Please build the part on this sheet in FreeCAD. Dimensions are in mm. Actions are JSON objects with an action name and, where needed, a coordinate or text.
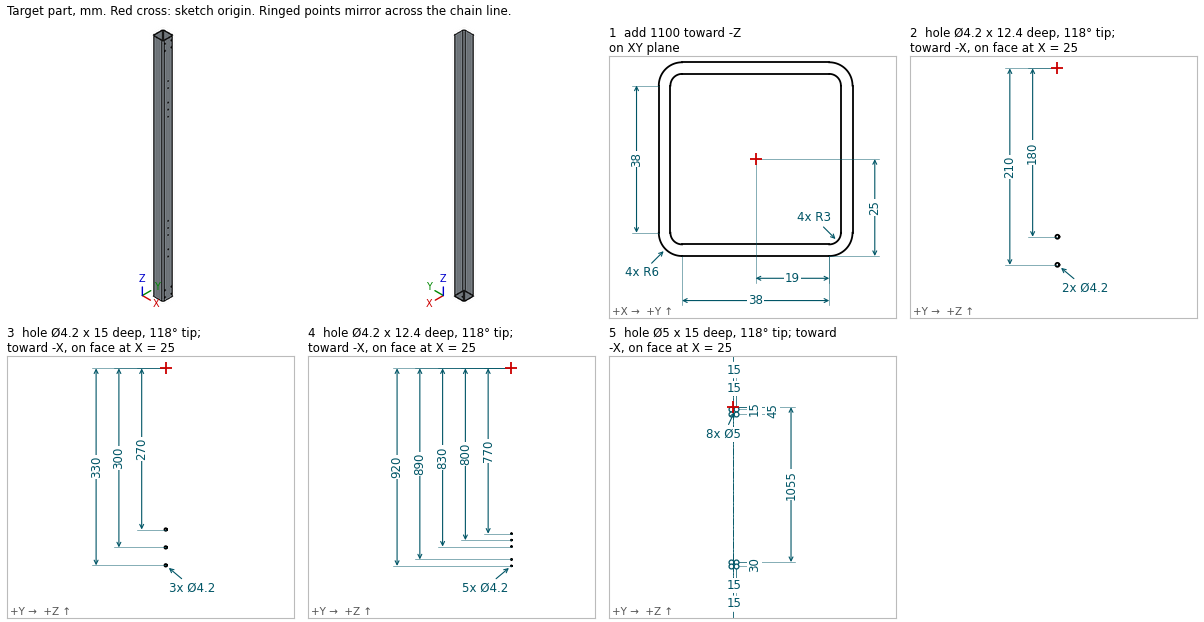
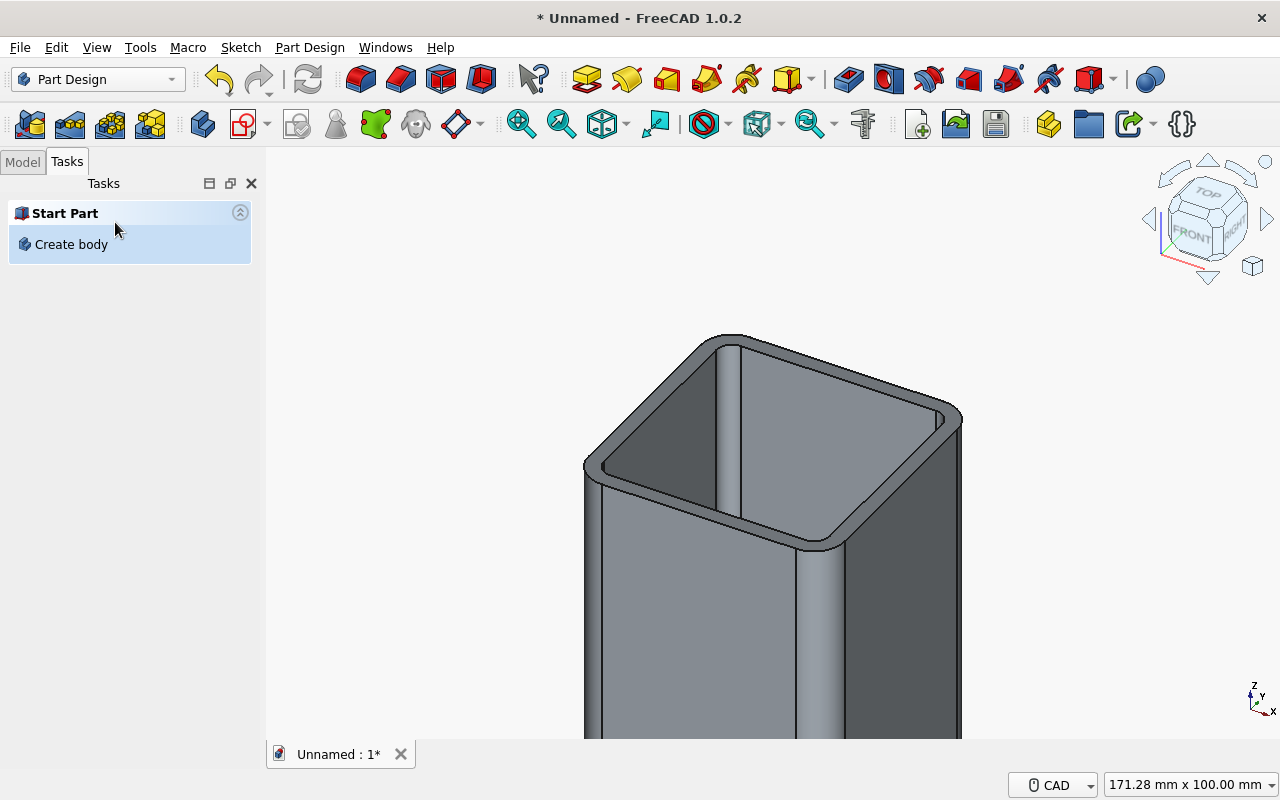
{"action": "left_click", "coordinate": [522, 124]}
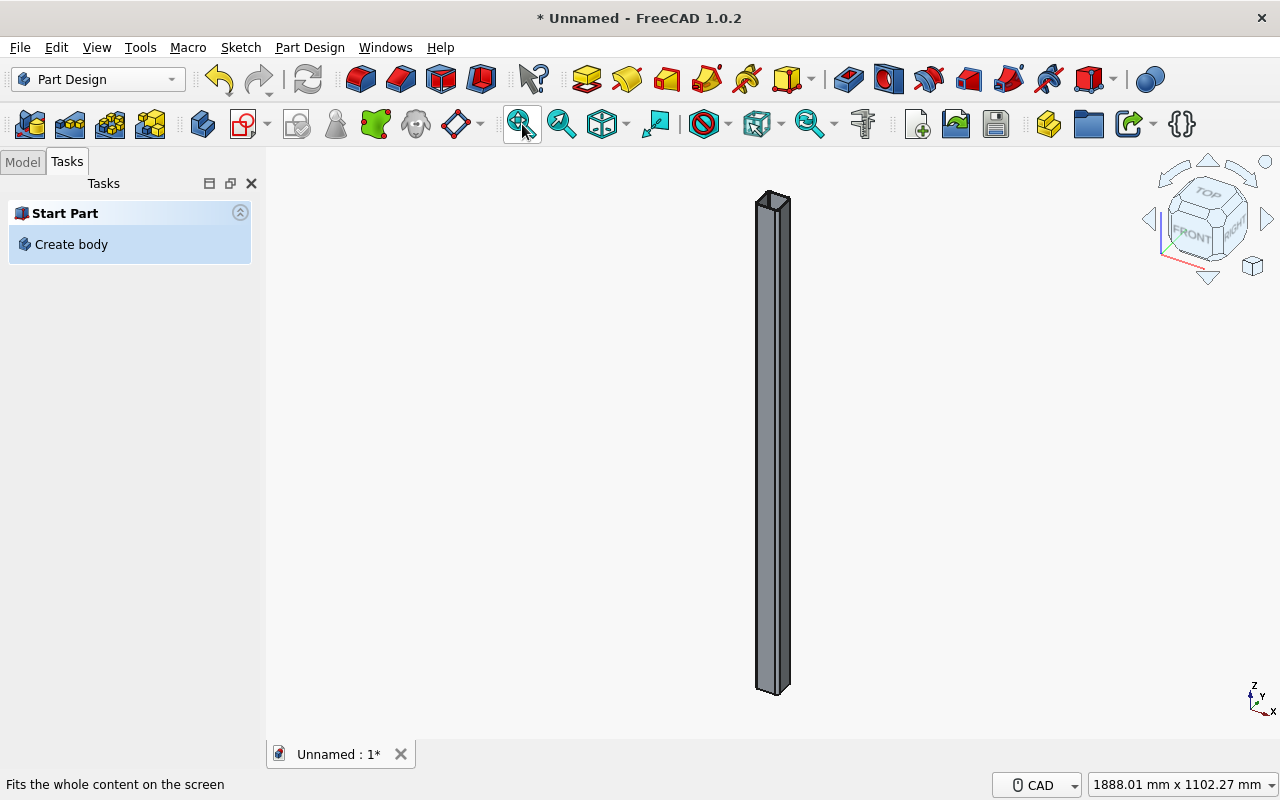
{"action": "key", "text": "0"}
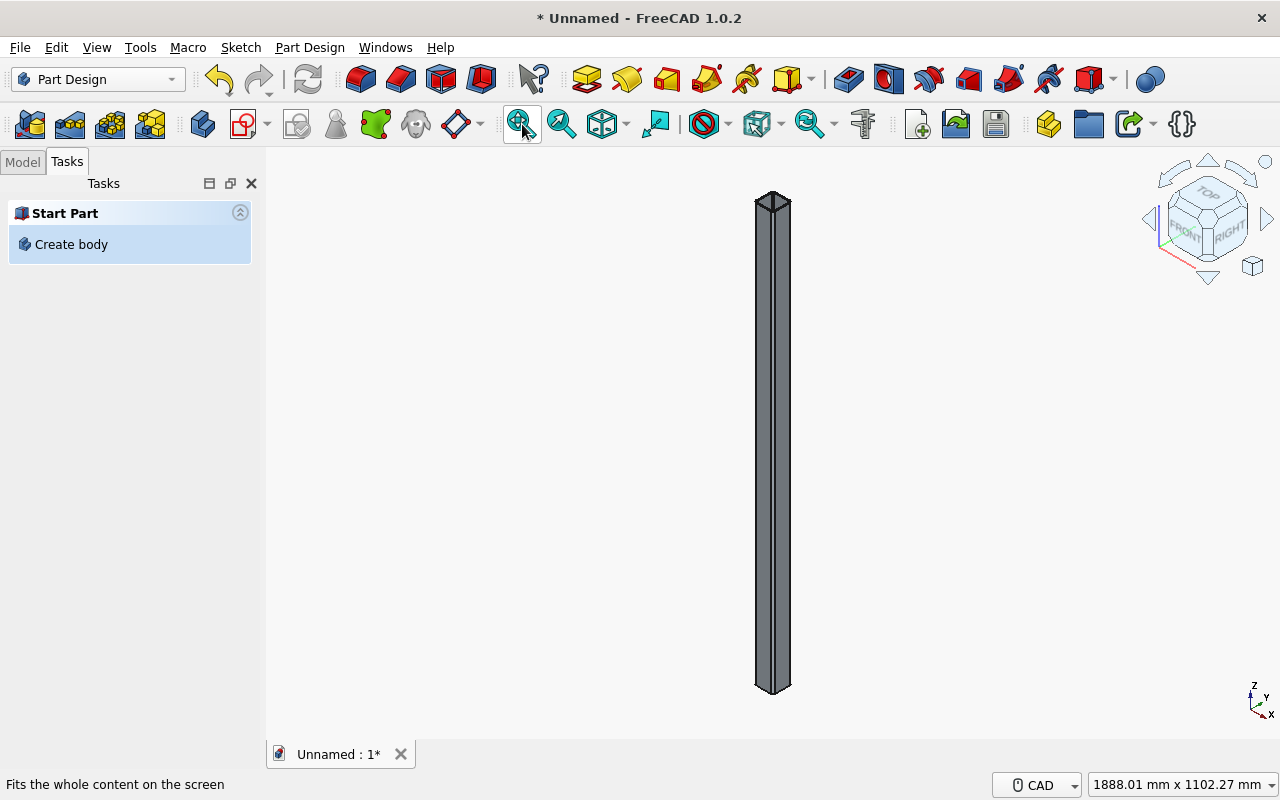
{"action": "left_click", "coordinate": [785, 240]}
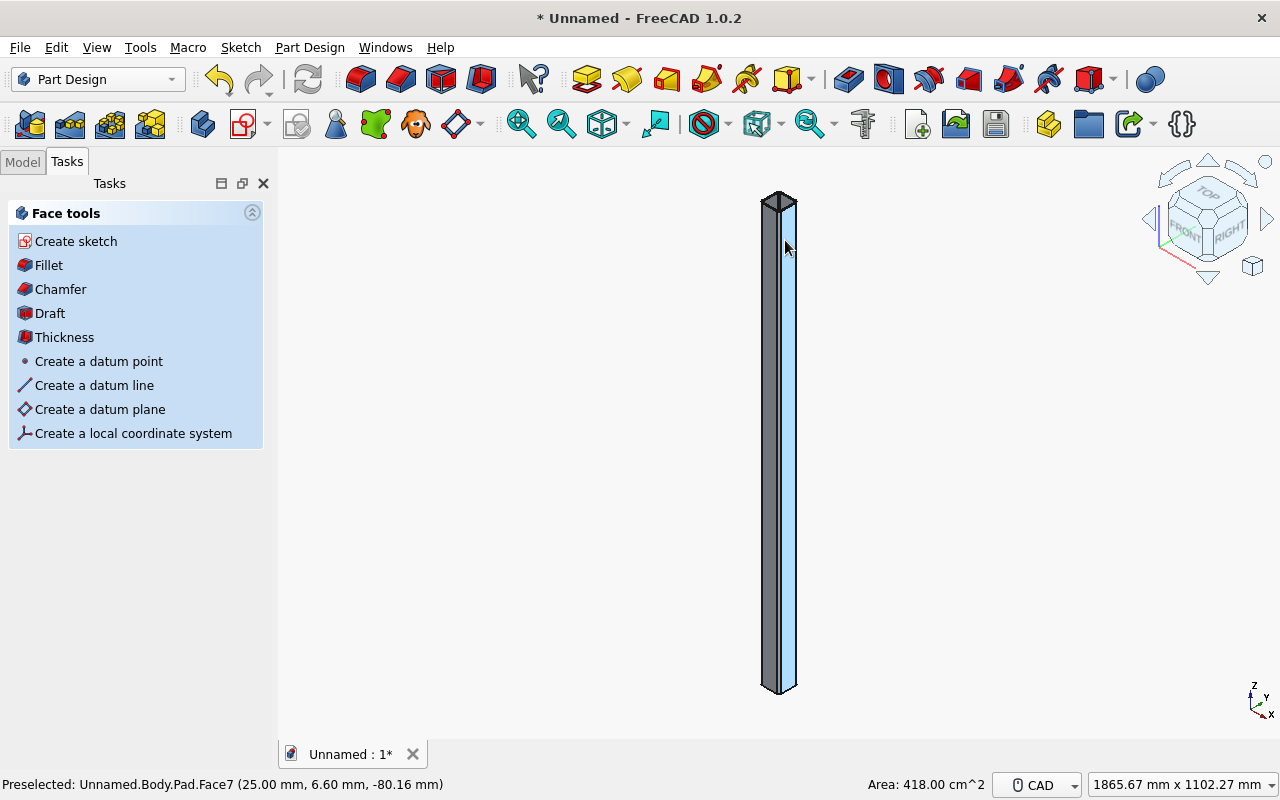
{"action": "left_click", "coordinate": [244, 124]}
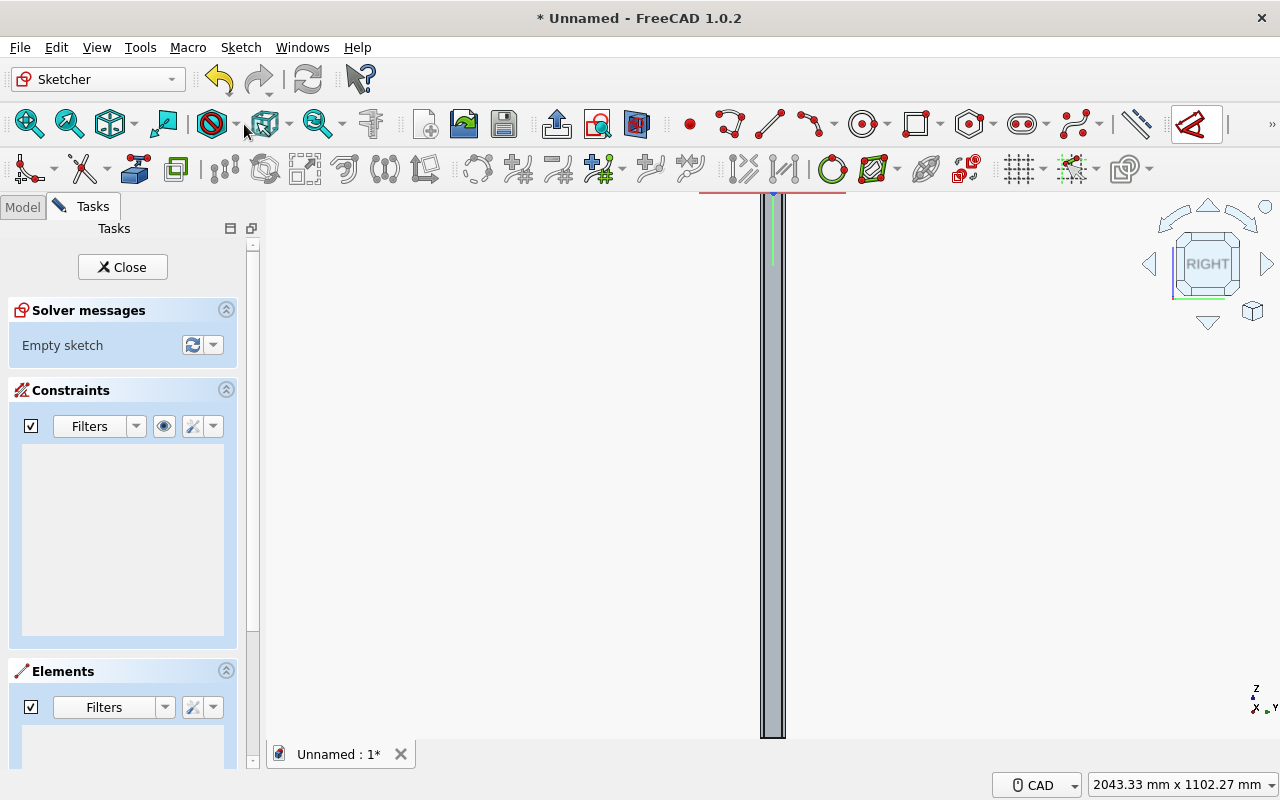
{"action": "scroll", "coordinate": [777, 280], "scroll_direction": "up", "scroll_amount": 15}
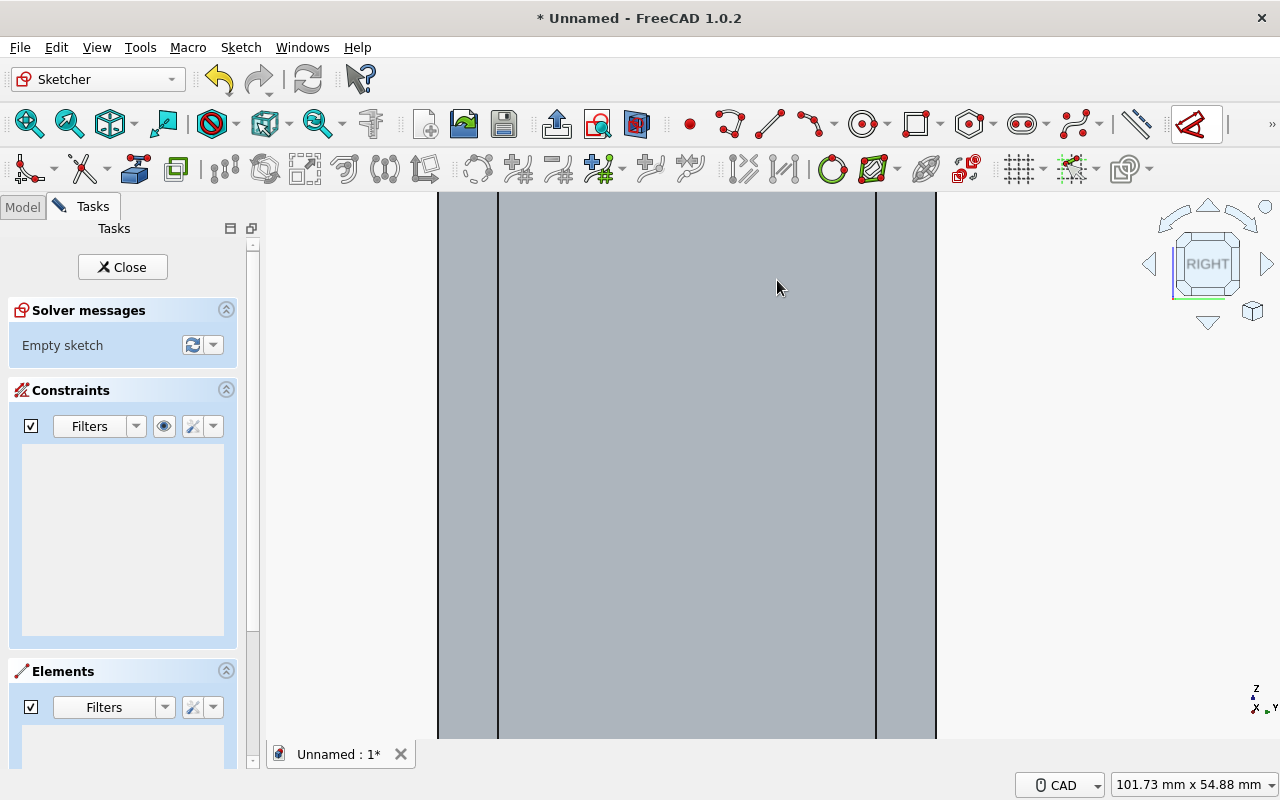
{"action": "left_click", "coordinate": [864, 124]}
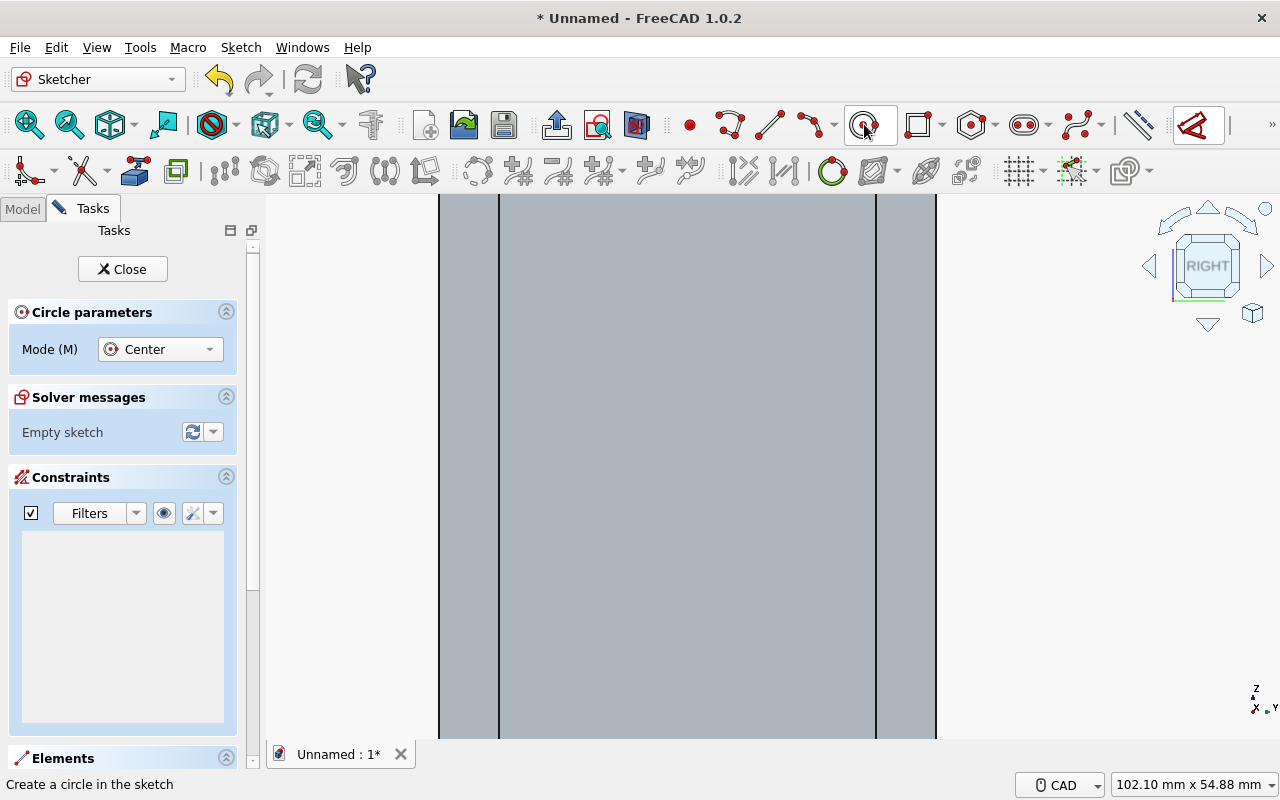
{"action": "left_click", "coordinate": [687, 316]}
{"action": "mouse_move", "coordinate": [702, 302]}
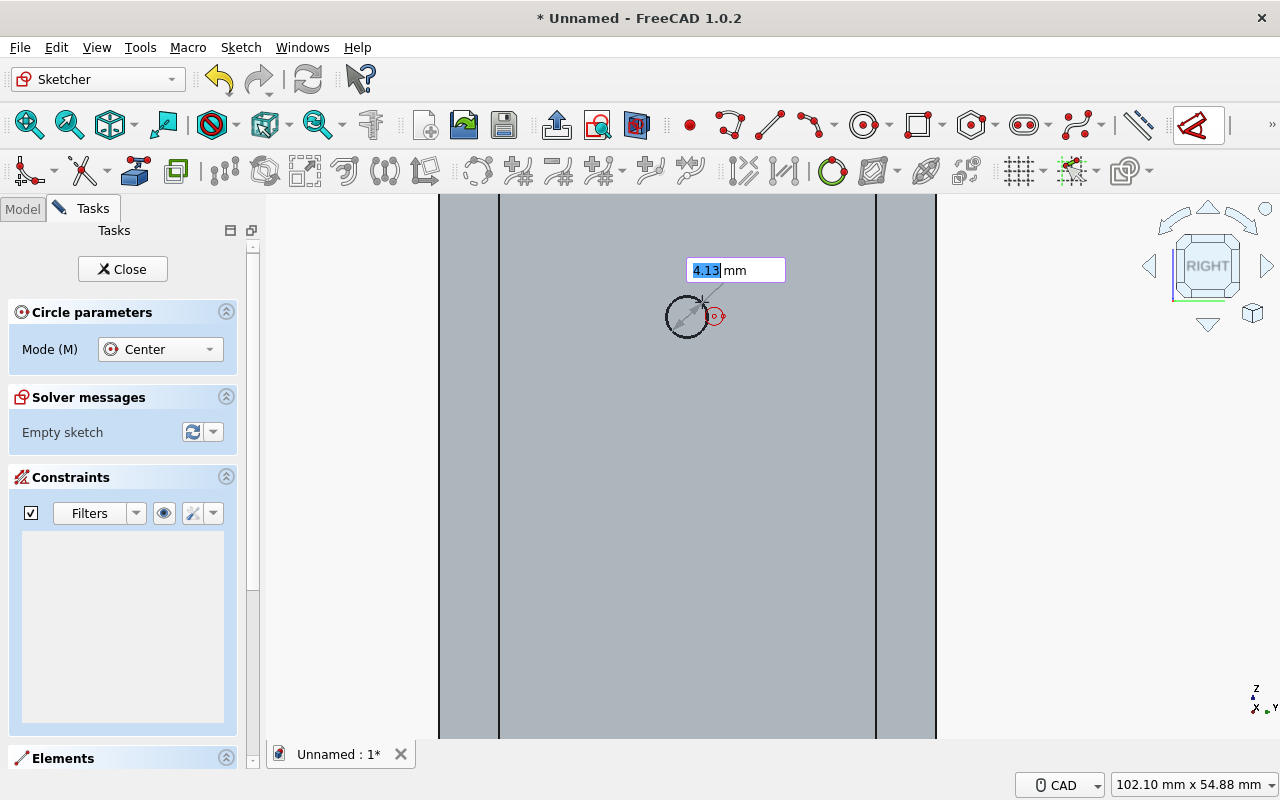
{"action": "type", "text": "4.2"}
{"action": "key", "text": "Return"}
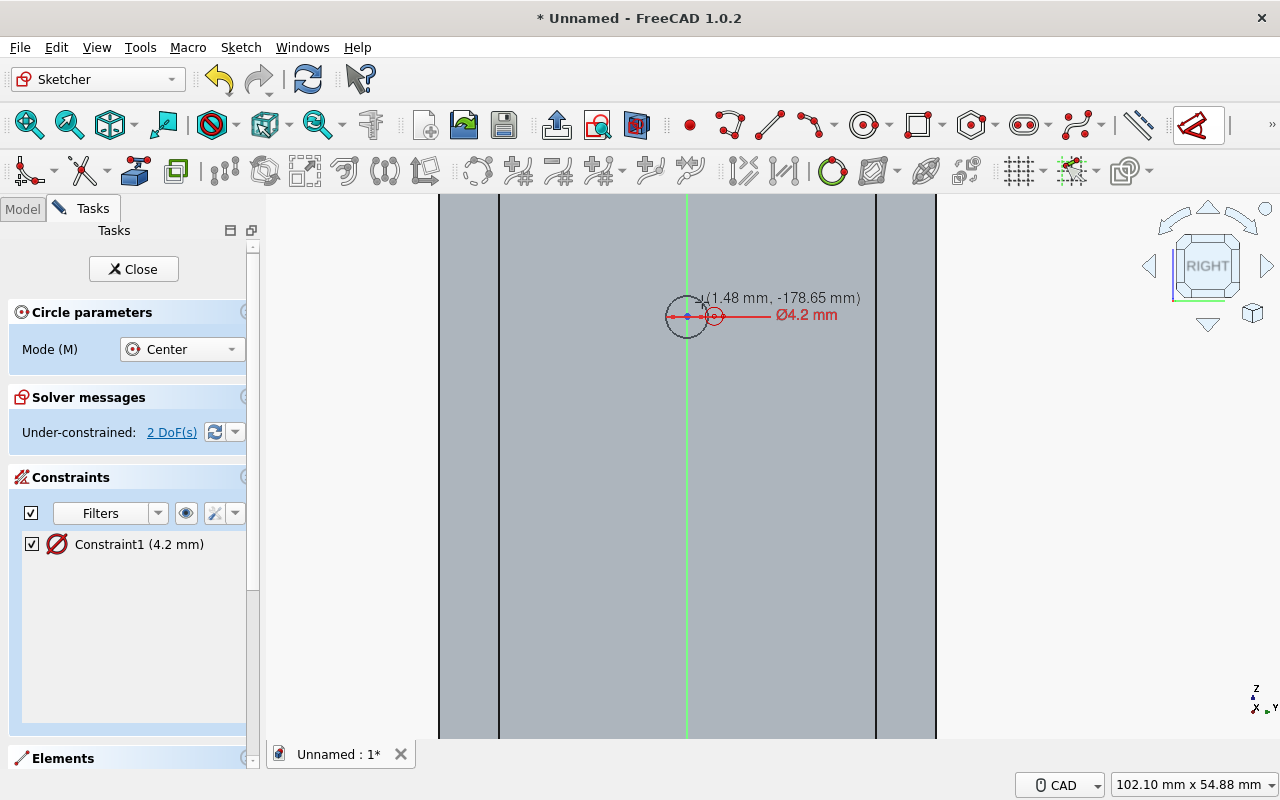
{"action": "left_click", "coordinate": [687, 614]}
{"action": "mouse_move", "coordinate": [702, 600]}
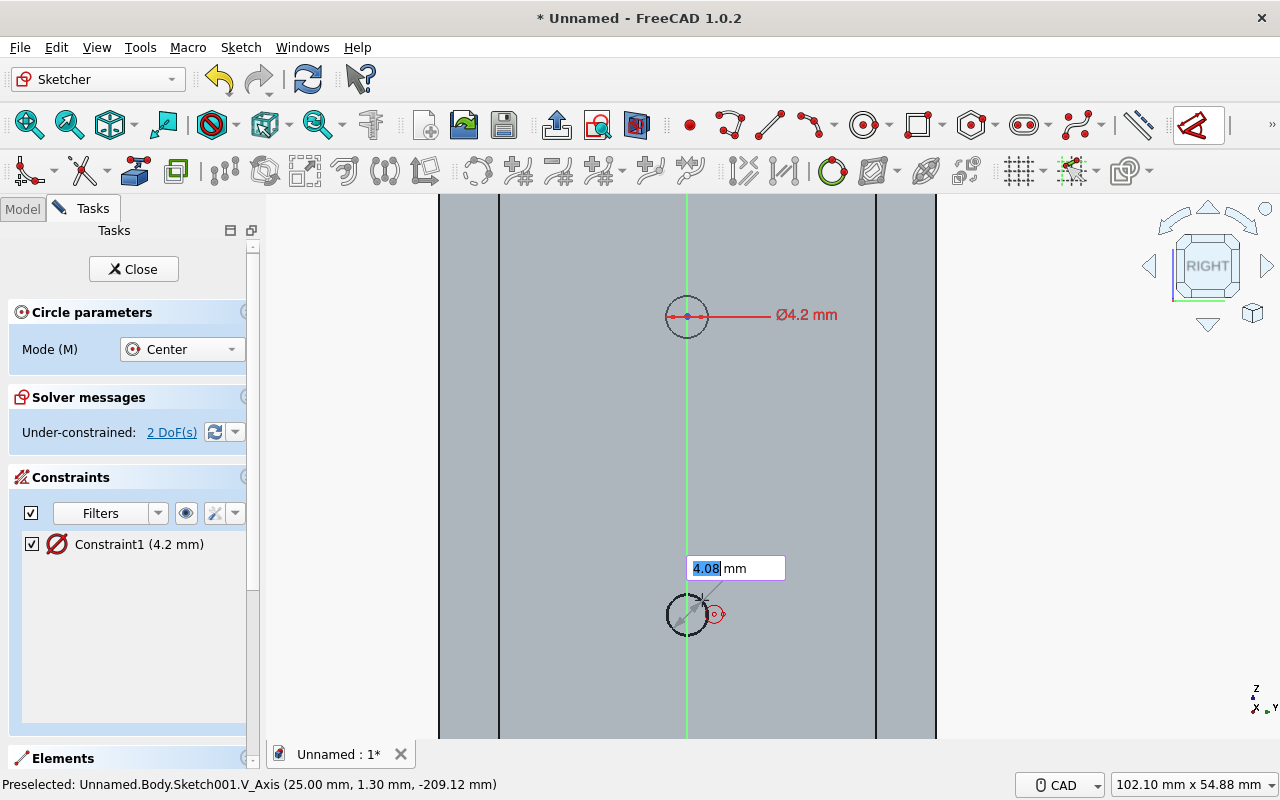
{"action": "type", "text": "4.2"}
{"action": "key", "text": "Return"}
{"action": "key", "text": "Escape"}